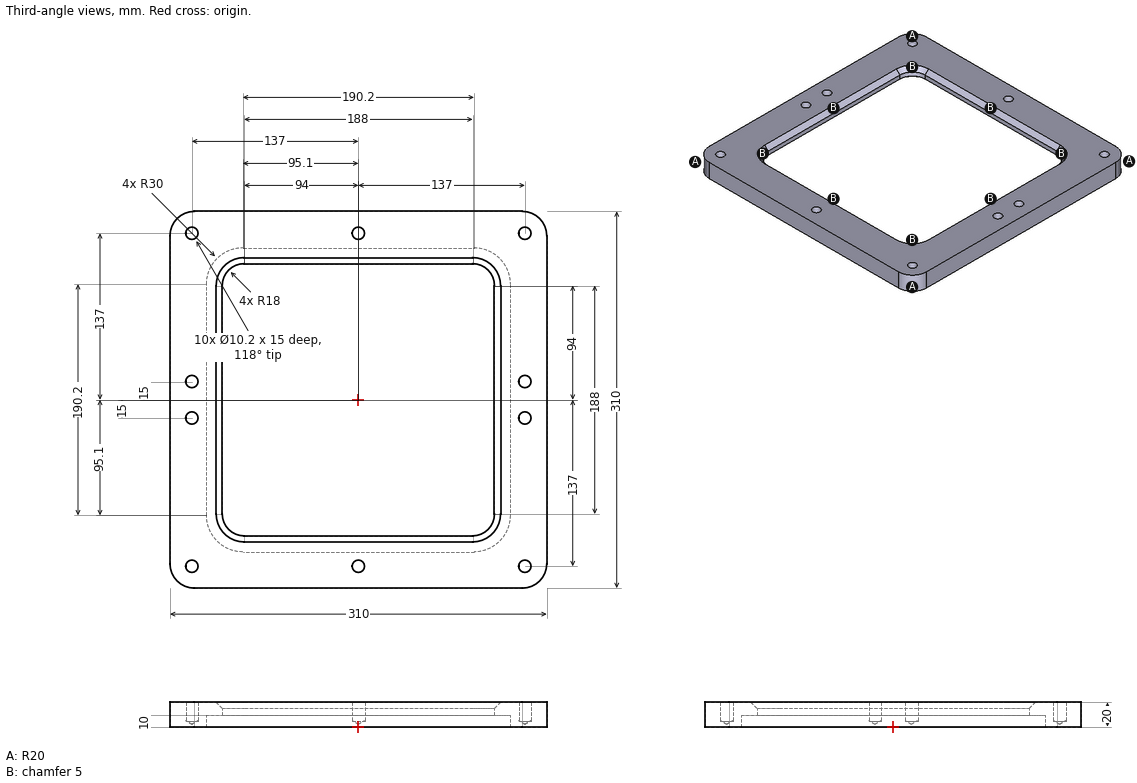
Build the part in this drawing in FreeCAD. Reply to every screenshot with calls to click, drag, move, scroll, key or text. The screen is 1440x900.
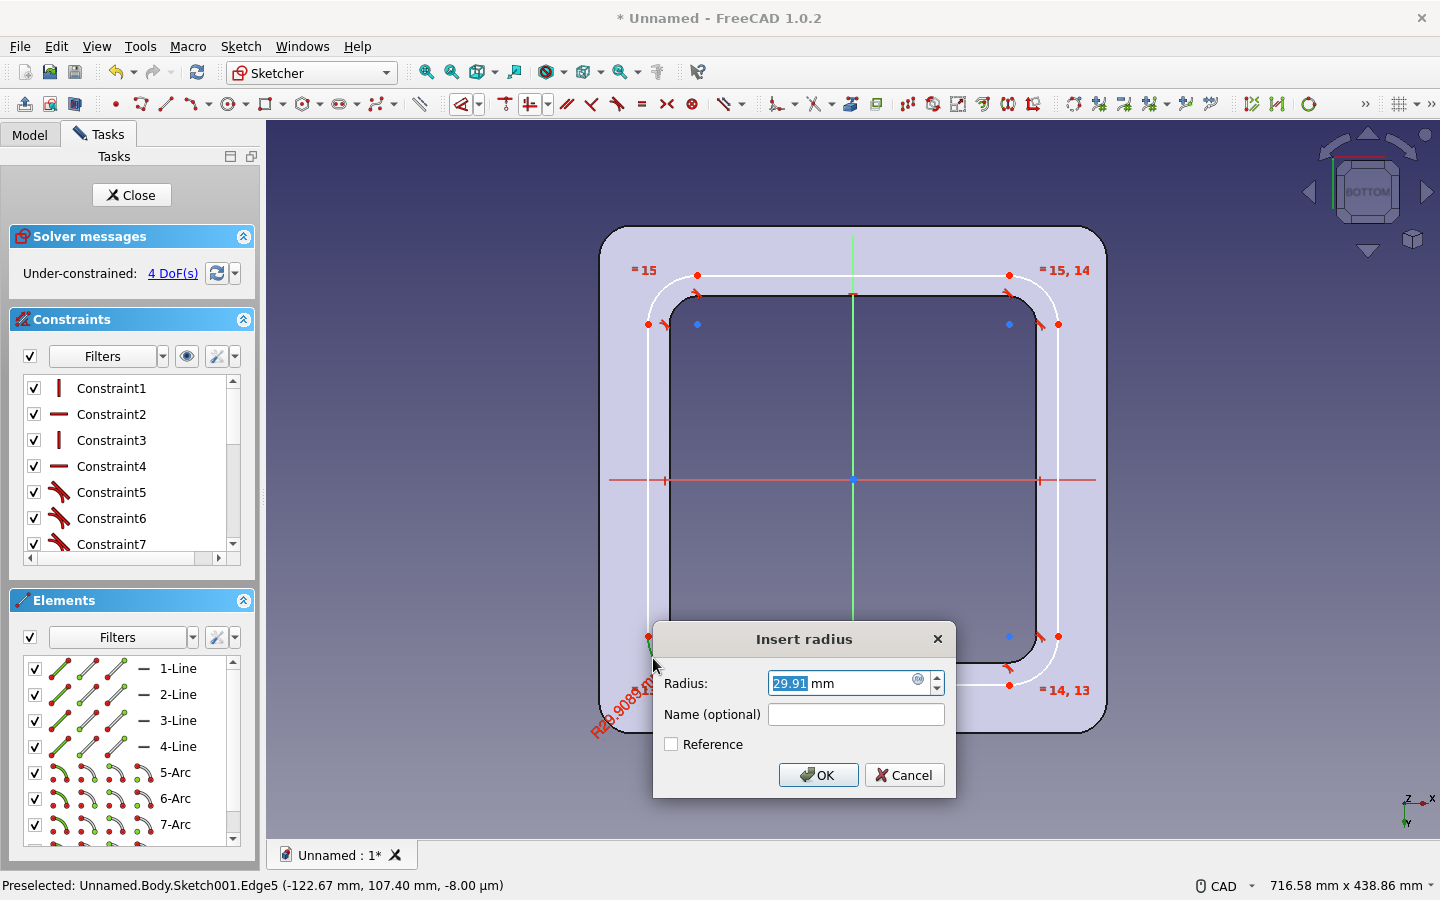
text(30)
key(Return)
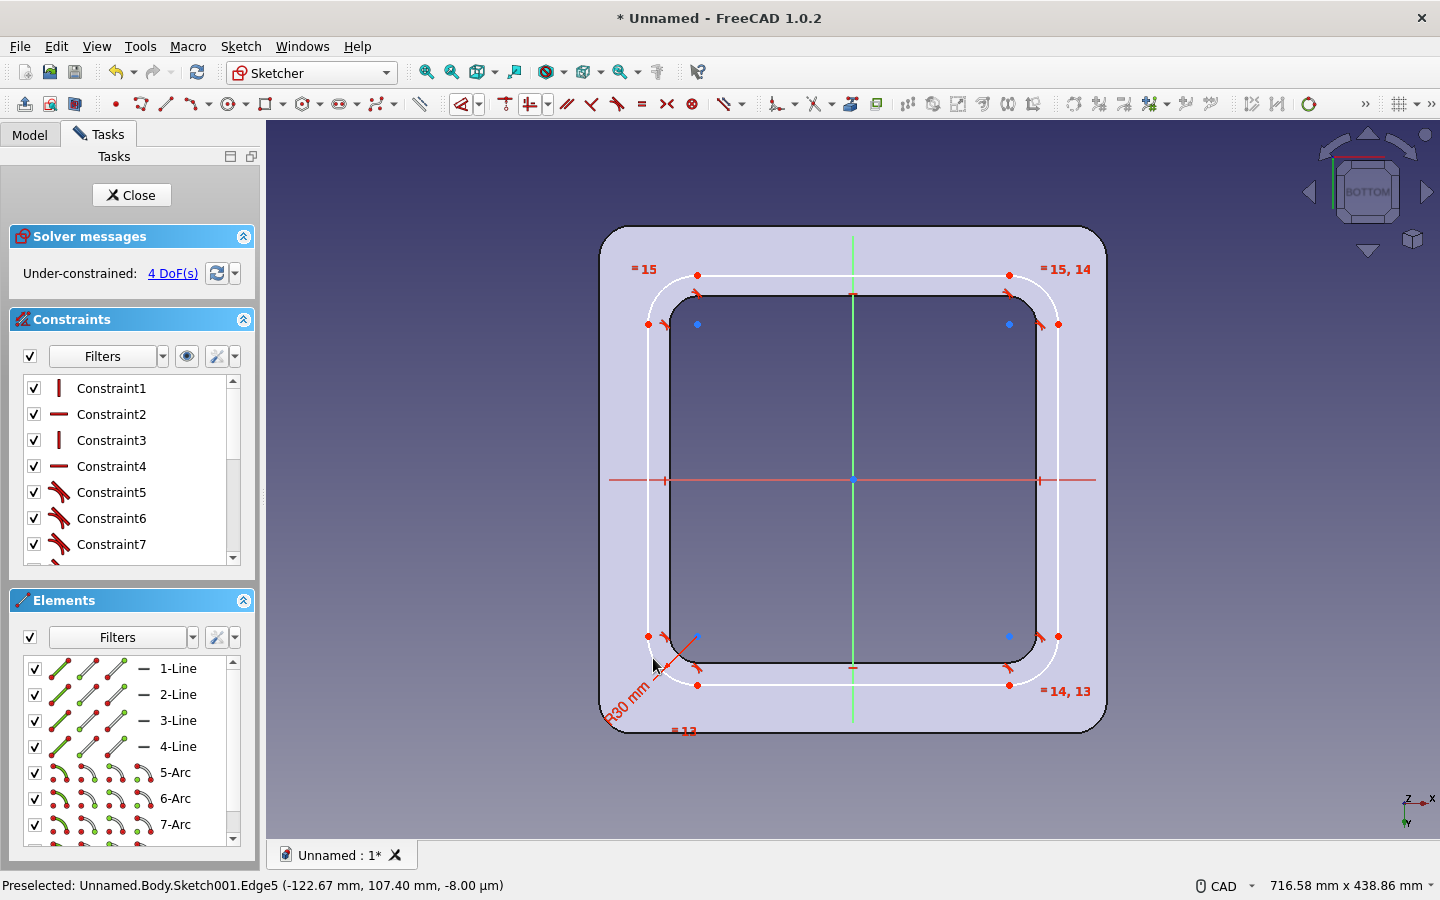
click(648, 418)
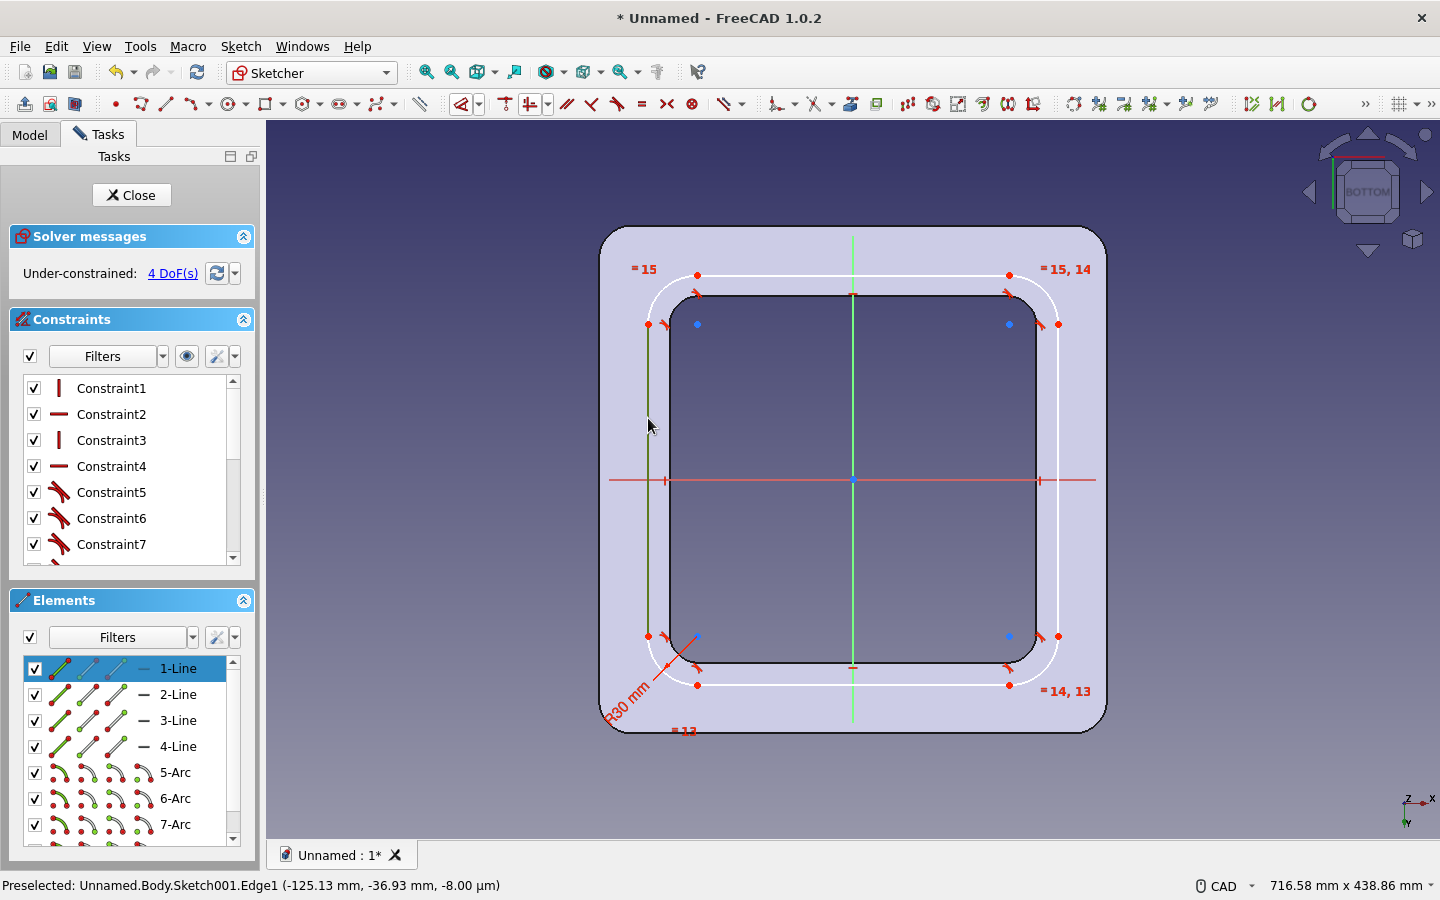
click(478, 104)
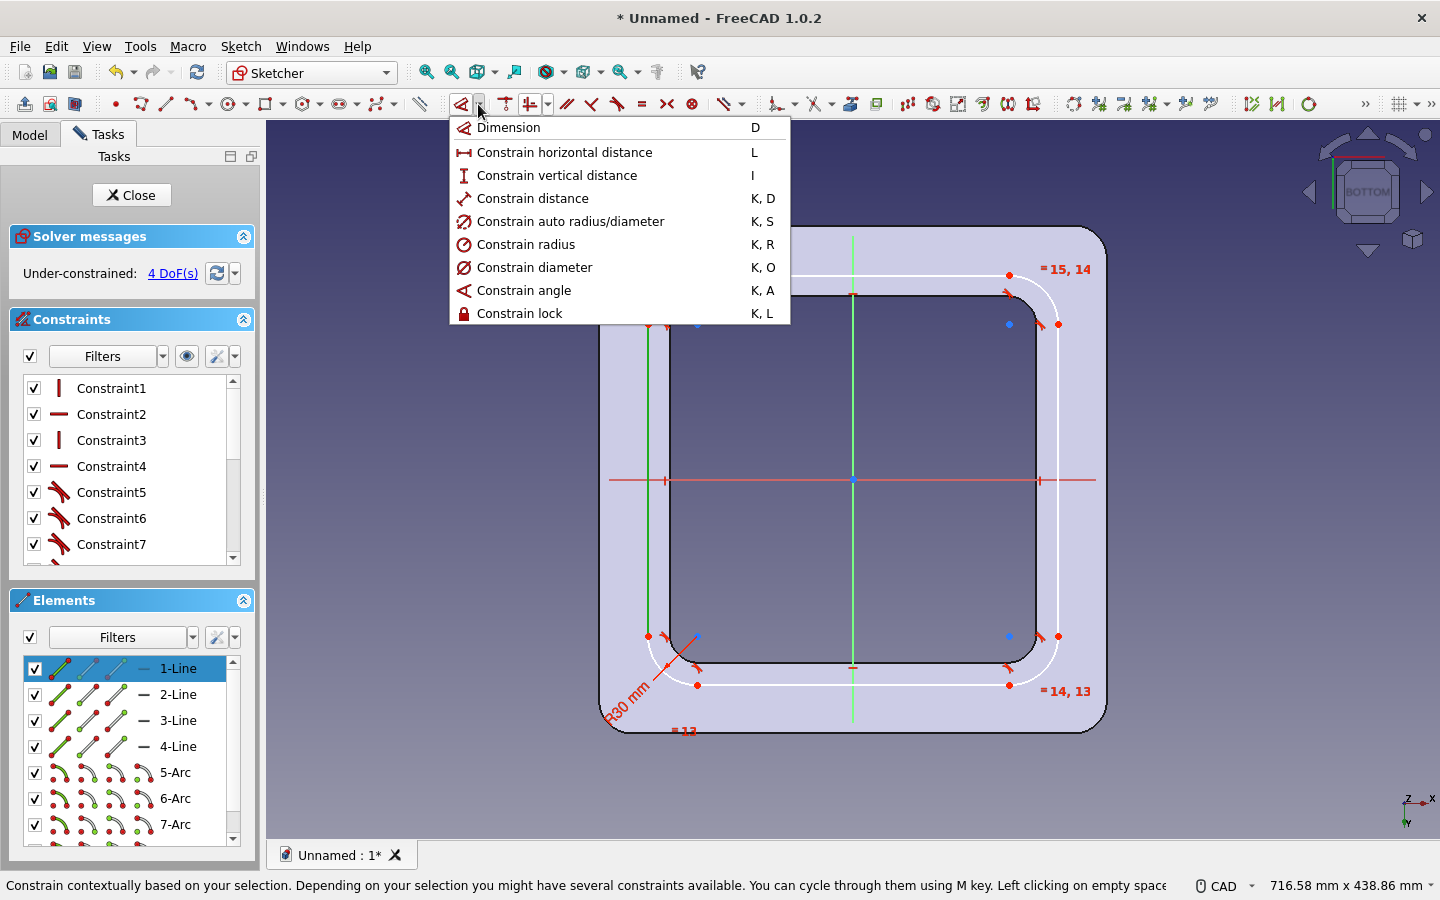
click(620, 176)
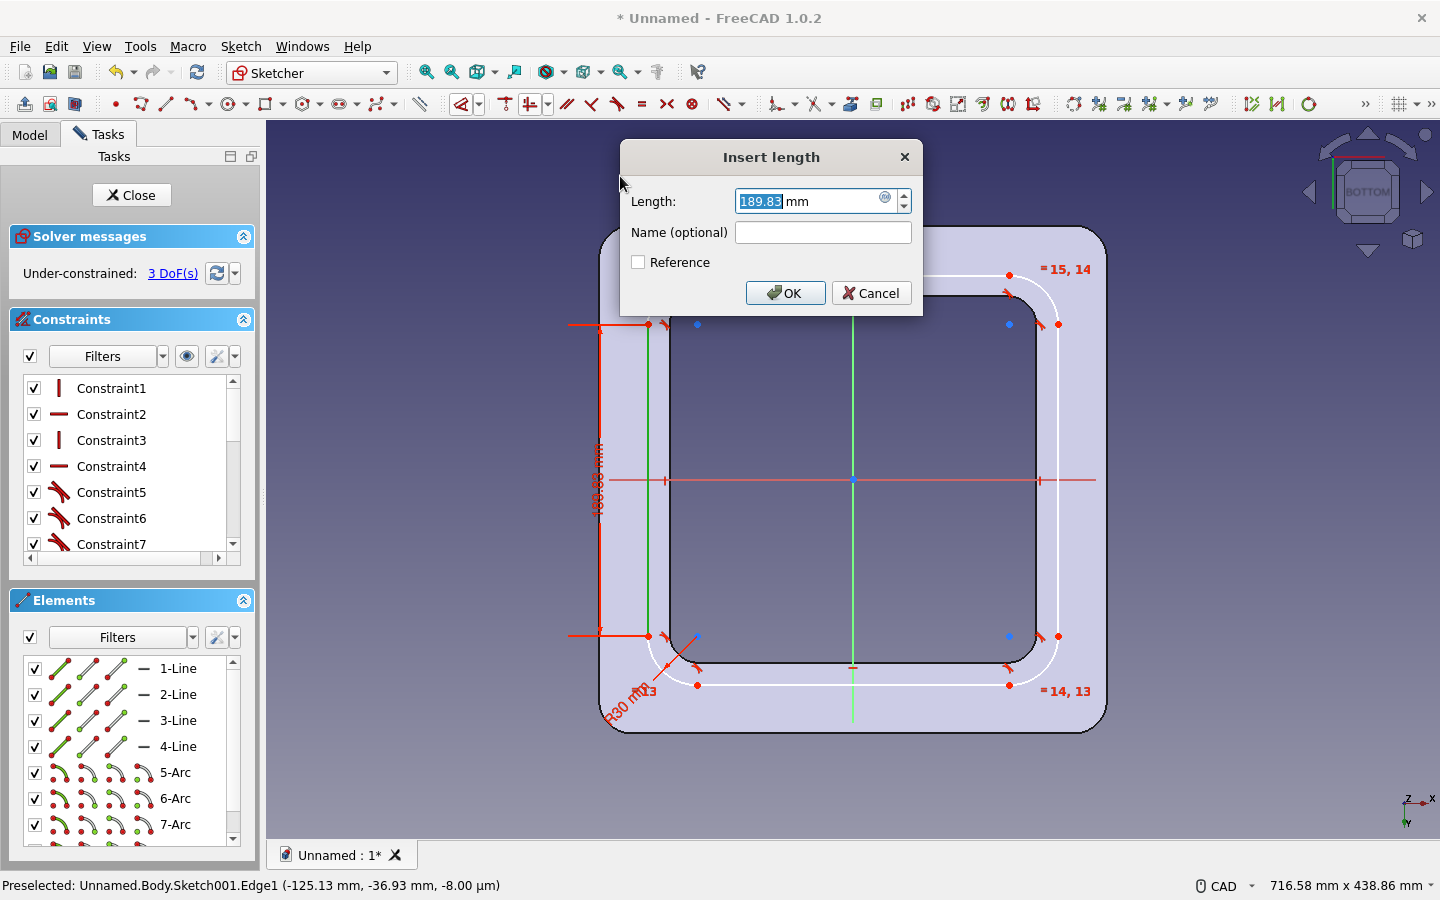
text(190.2)
key(Return)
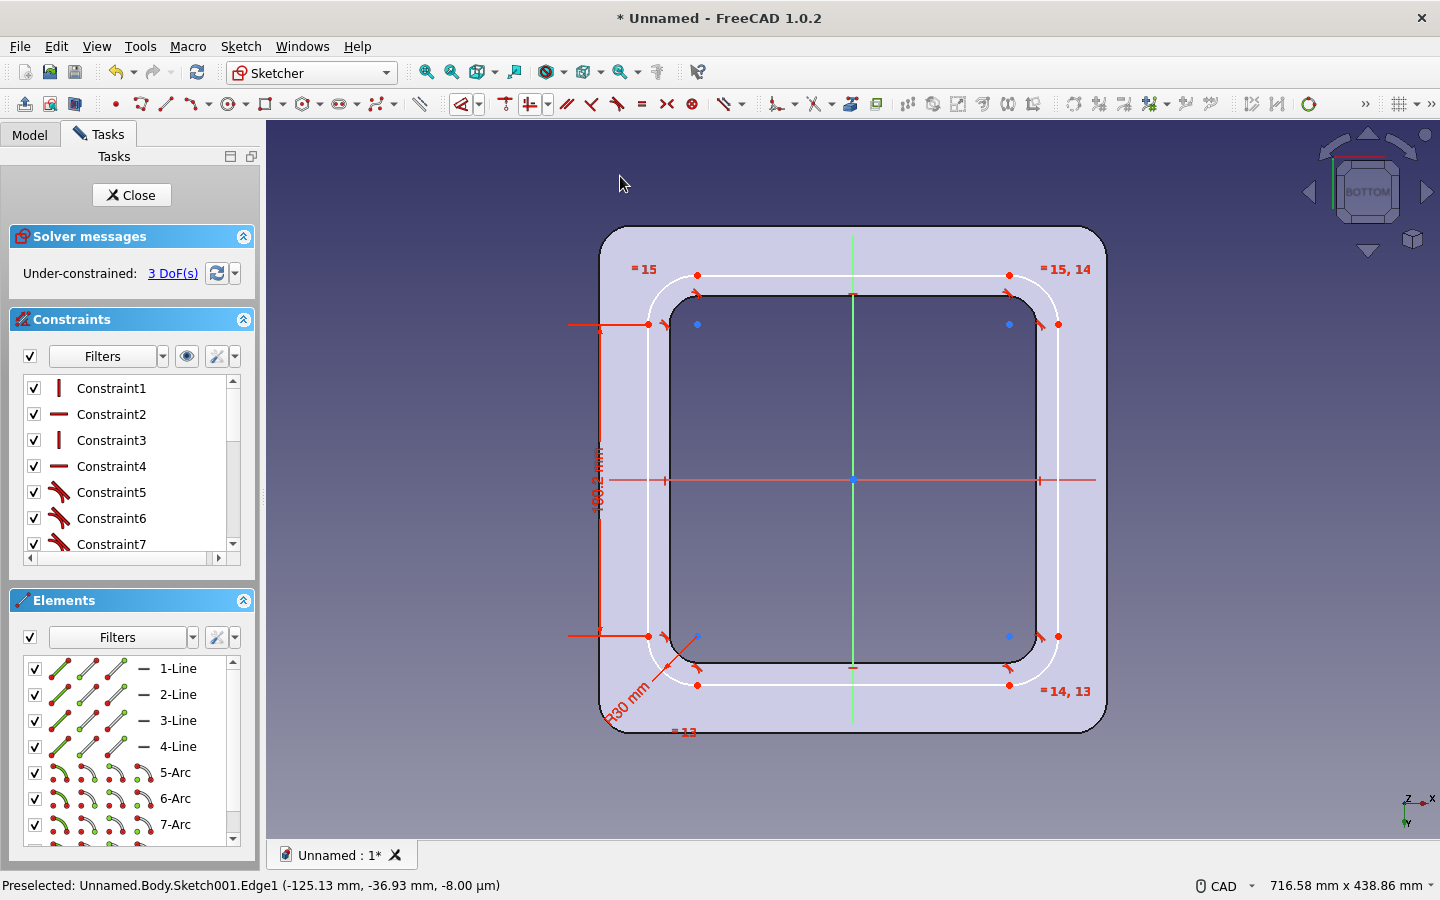
click(791, 685)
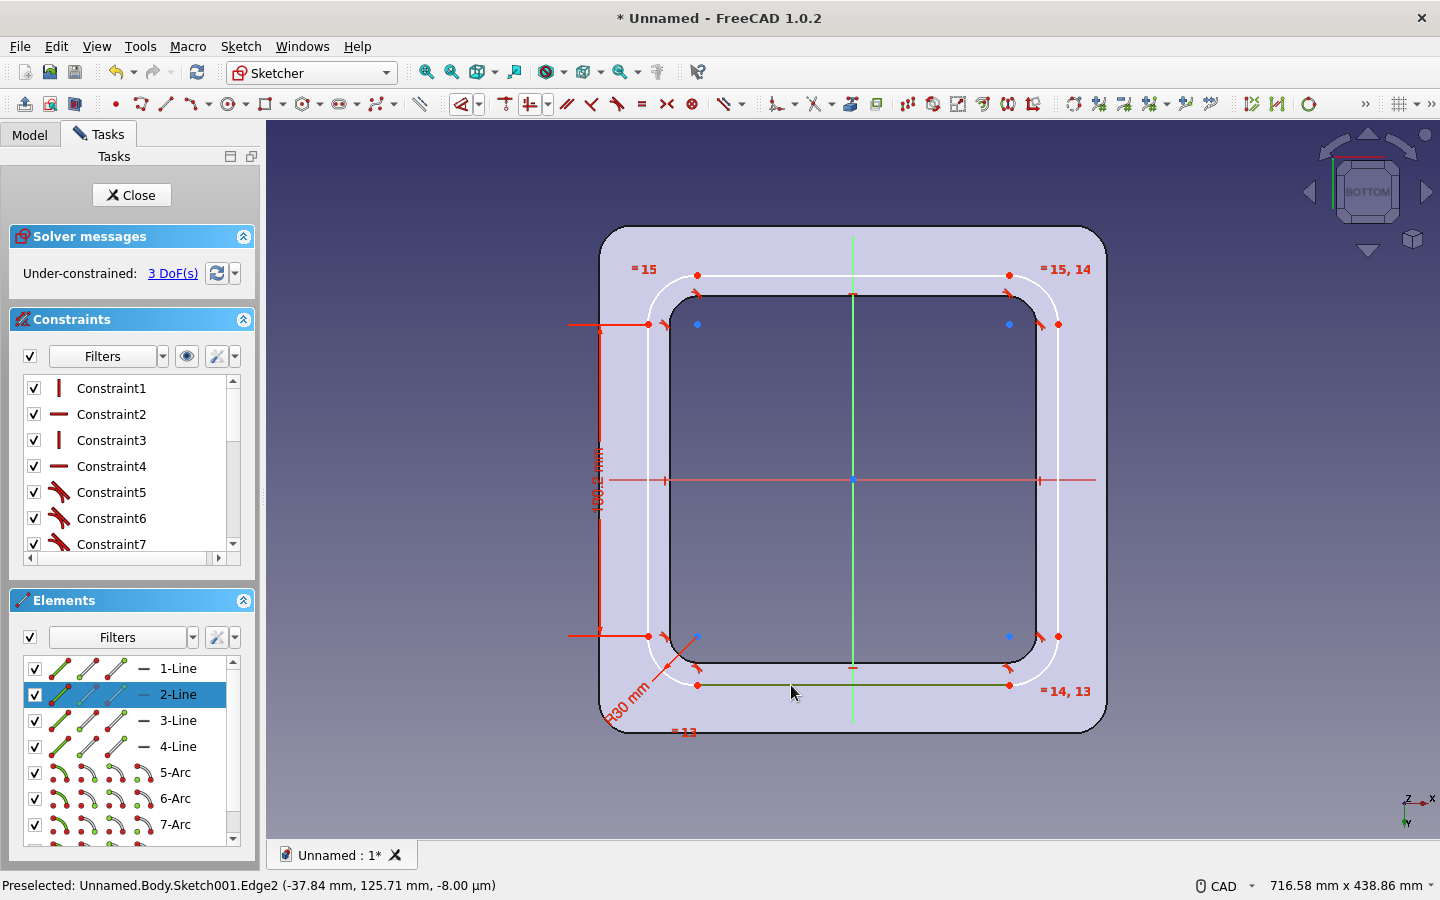
click(478, 104)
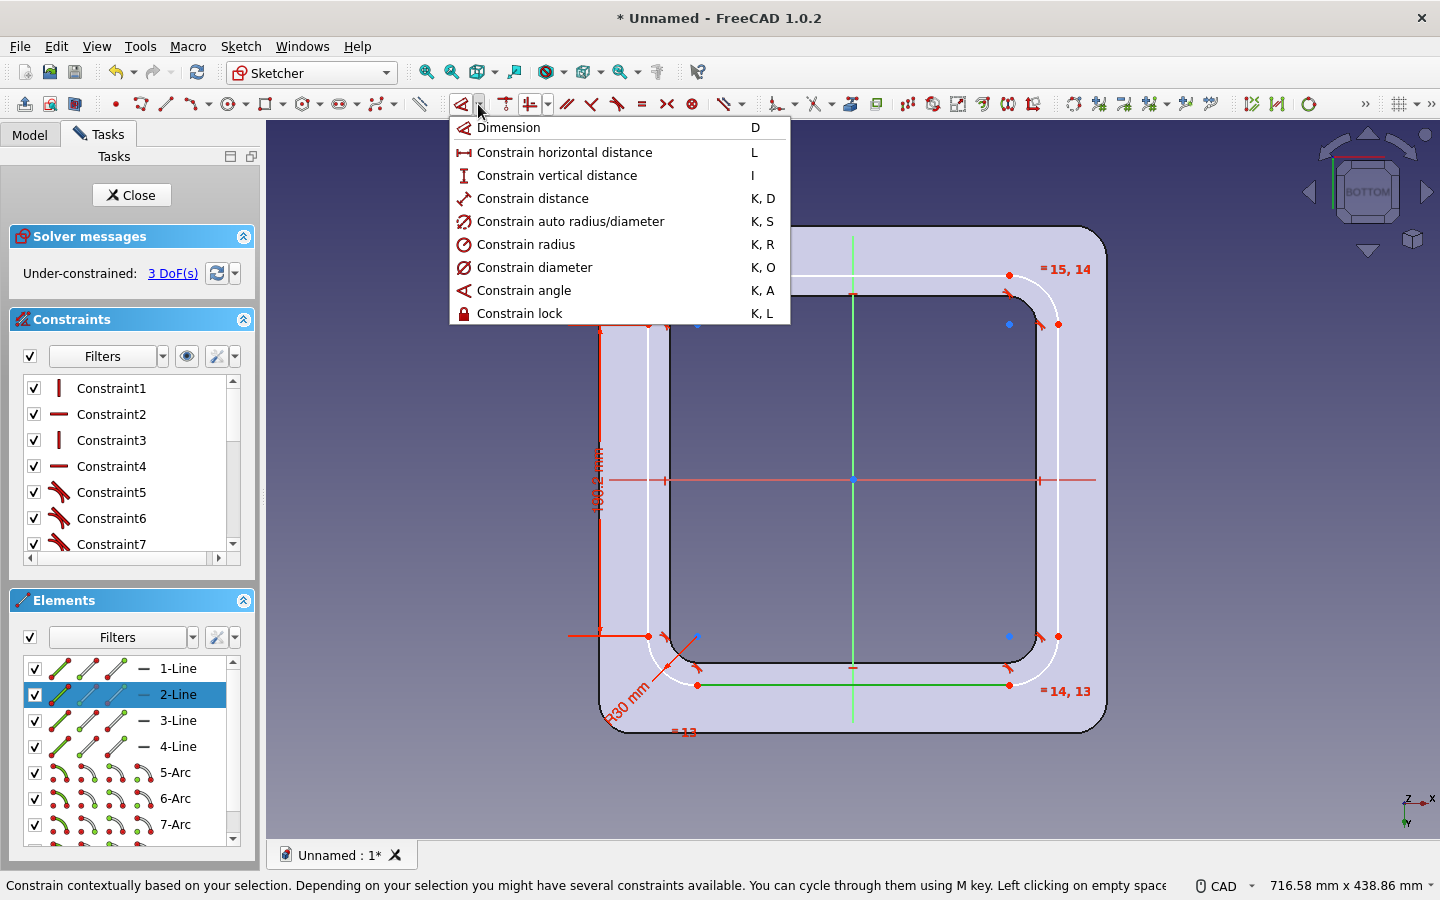
click(620, 152)